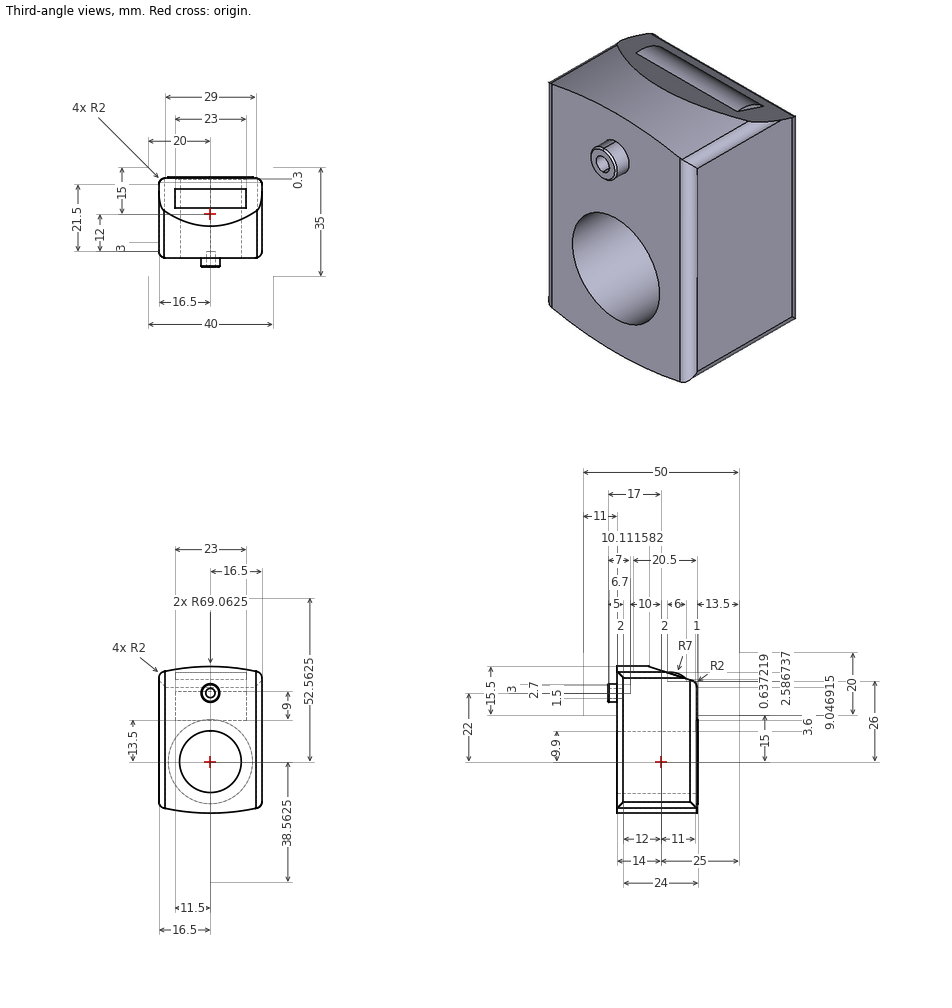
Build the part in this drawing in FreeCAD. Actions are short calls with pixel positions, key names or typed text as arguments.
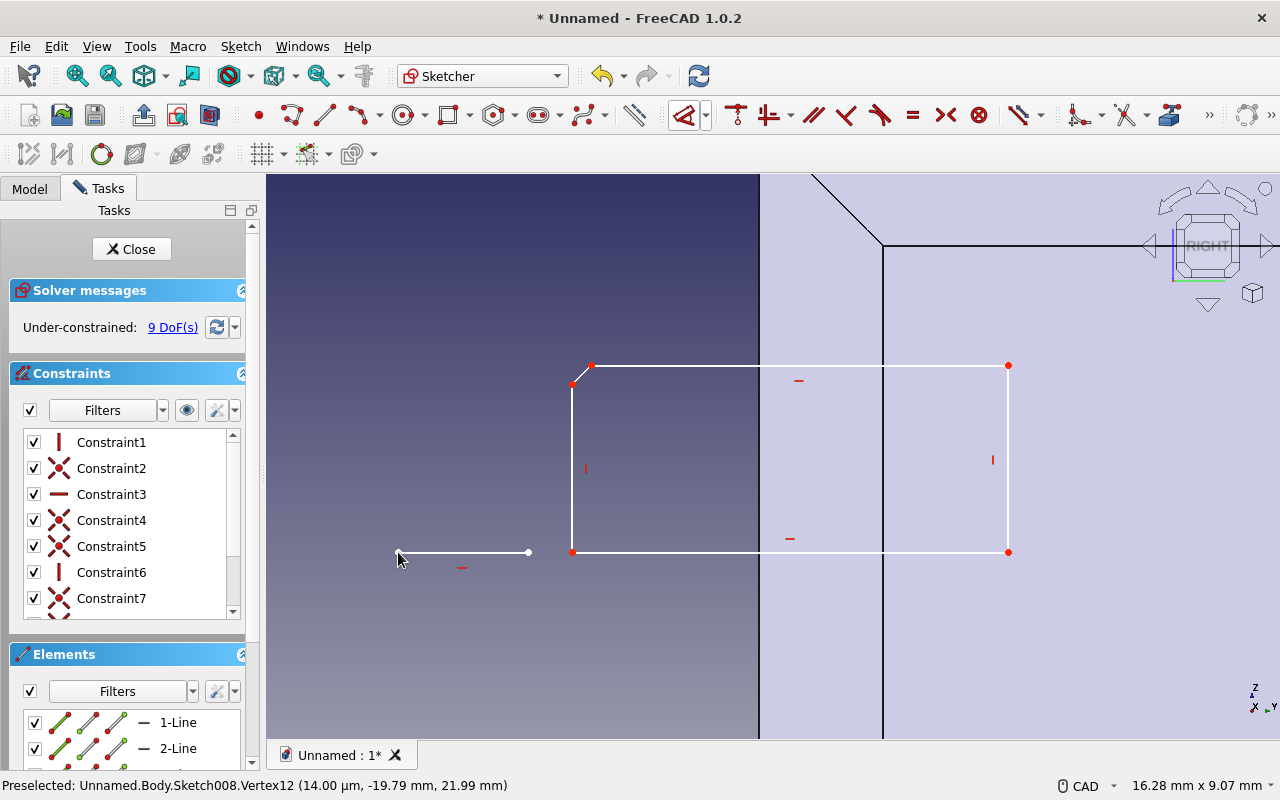
click(489, 553)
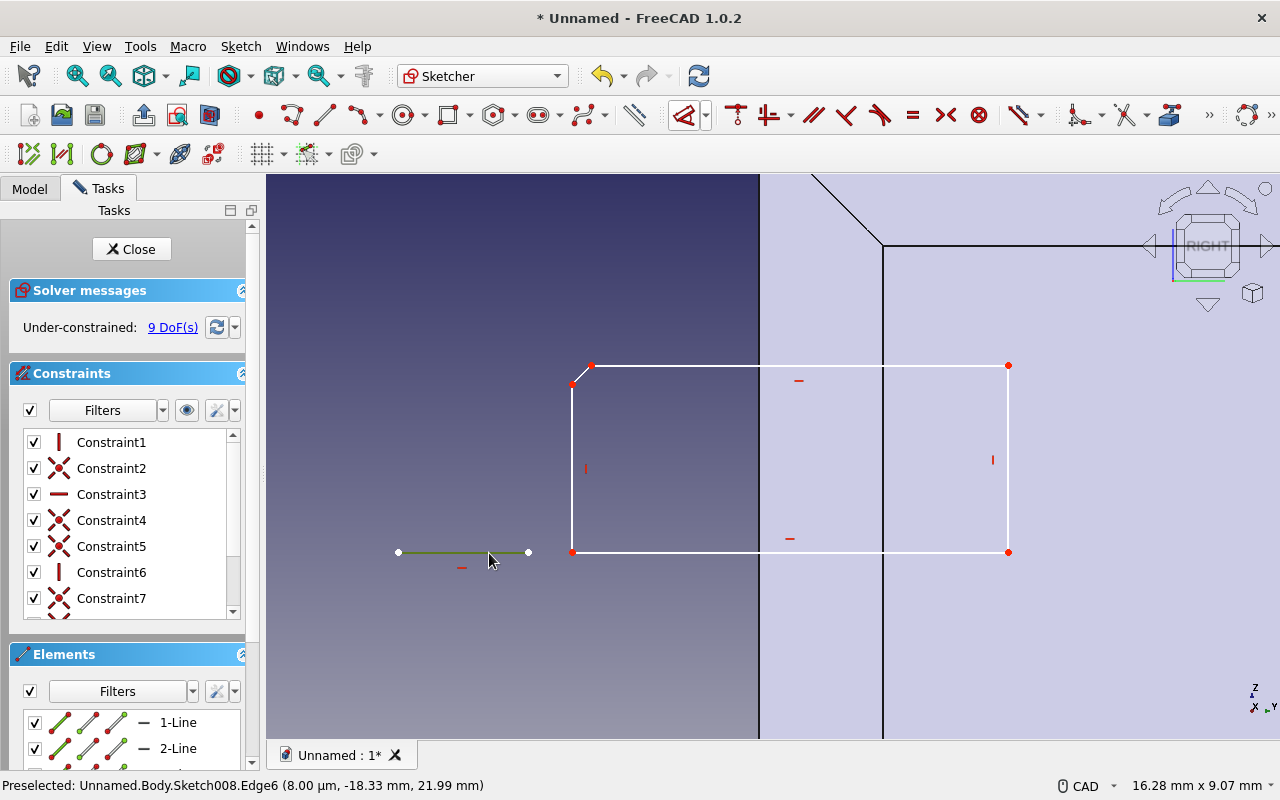
click(635, 116)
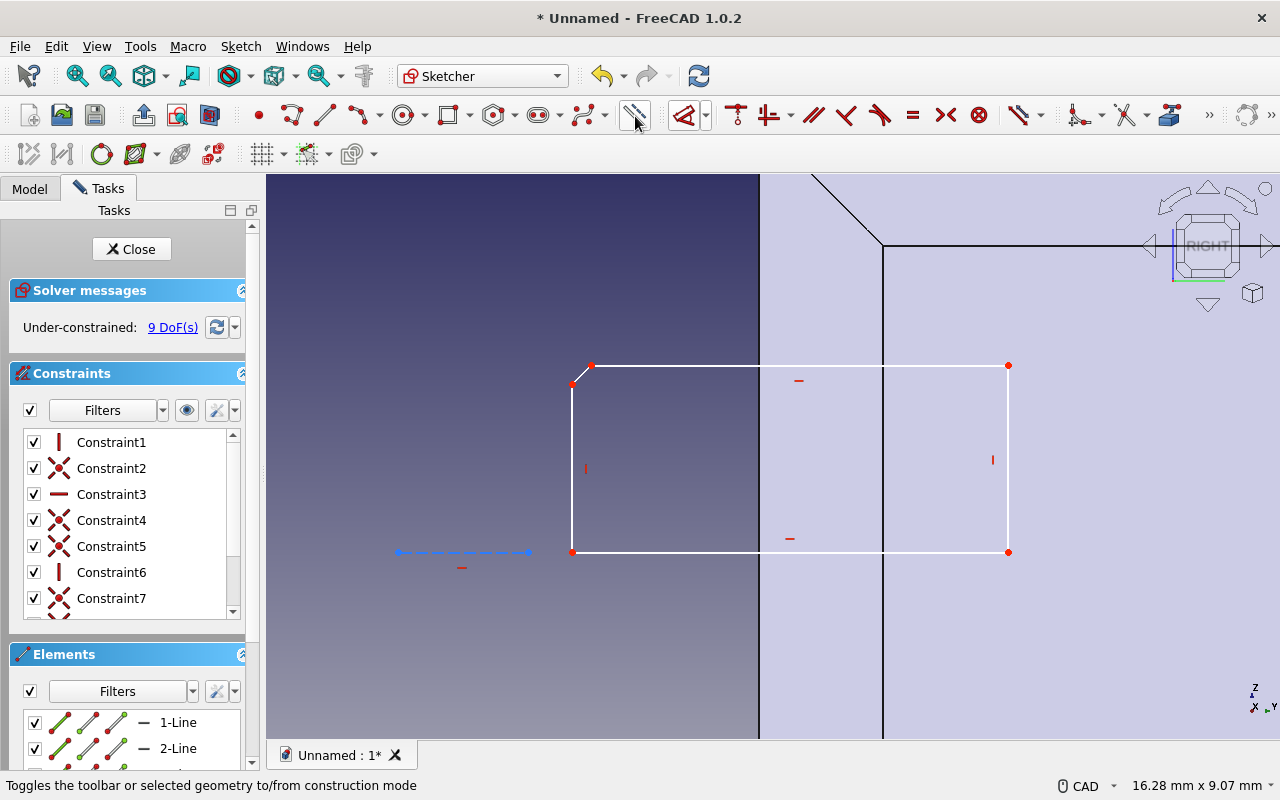
click(1008, 497)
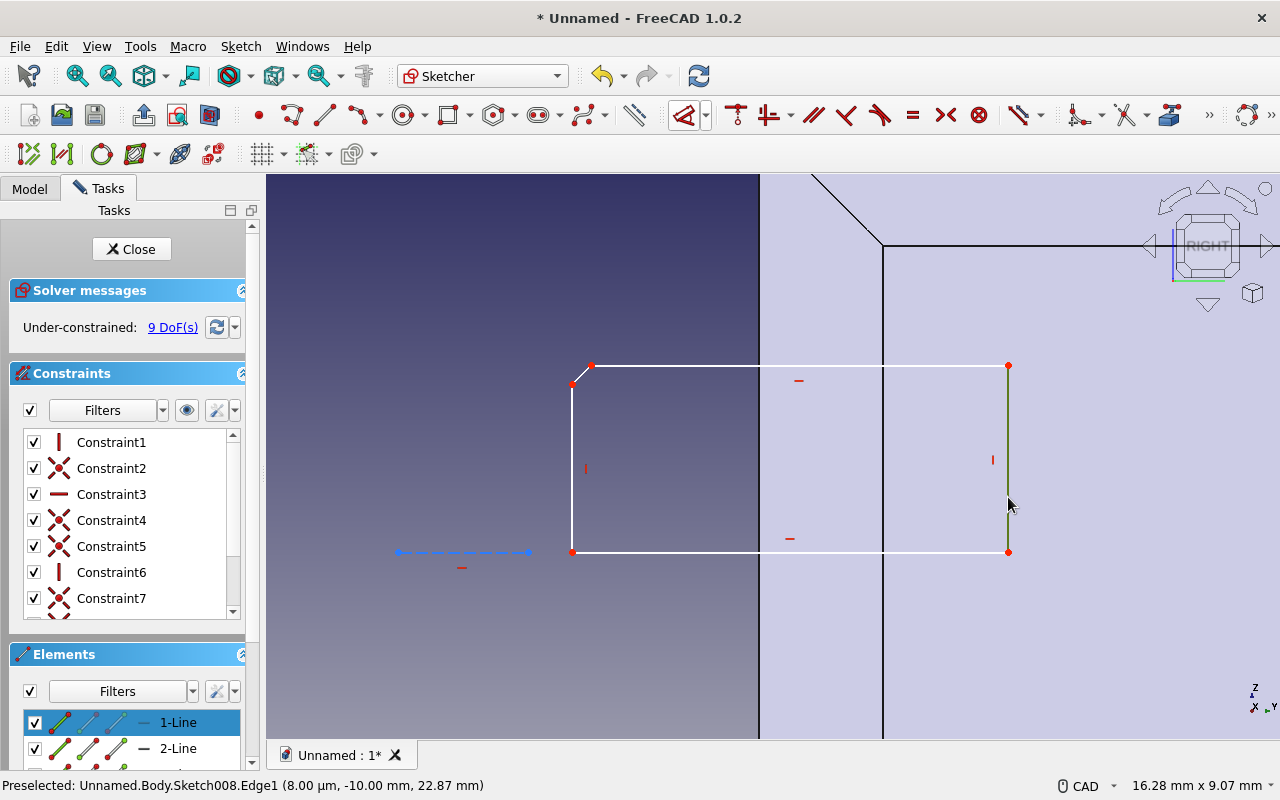
click(706, 116)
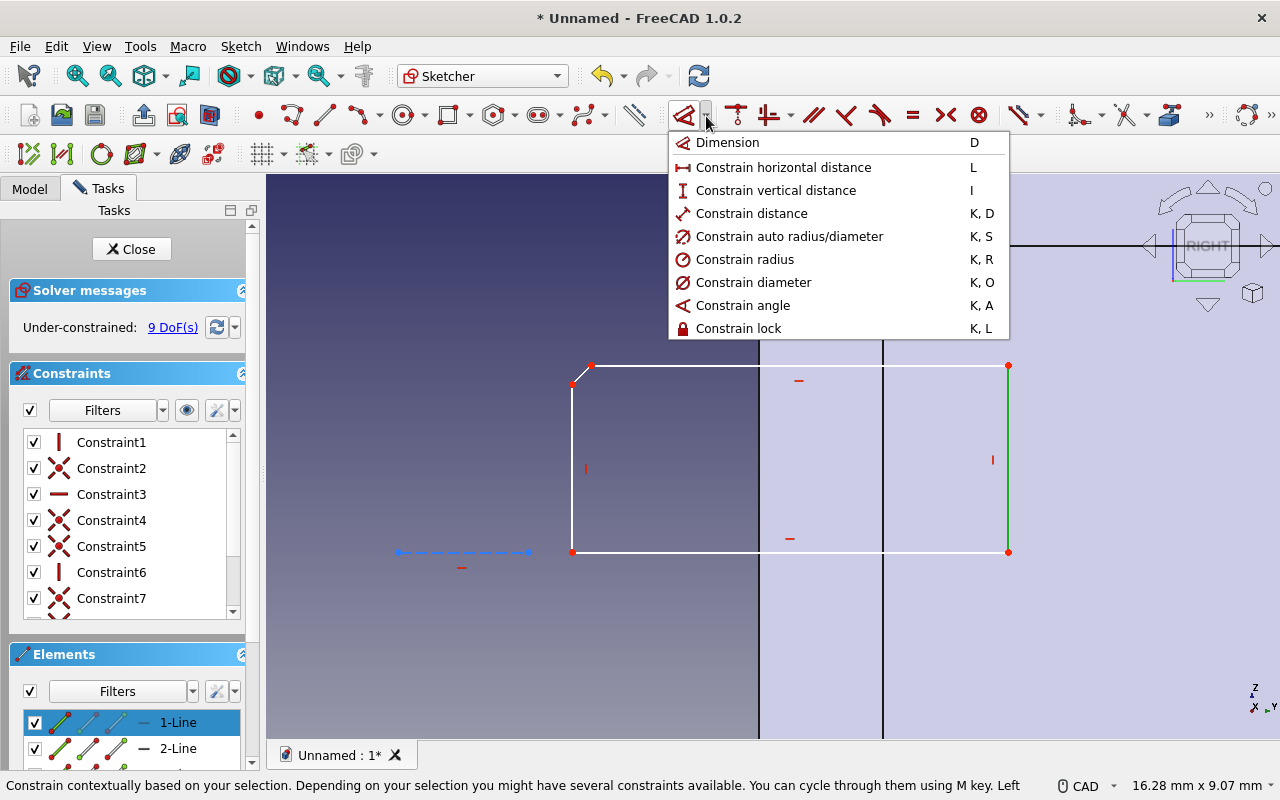
click(839, 190)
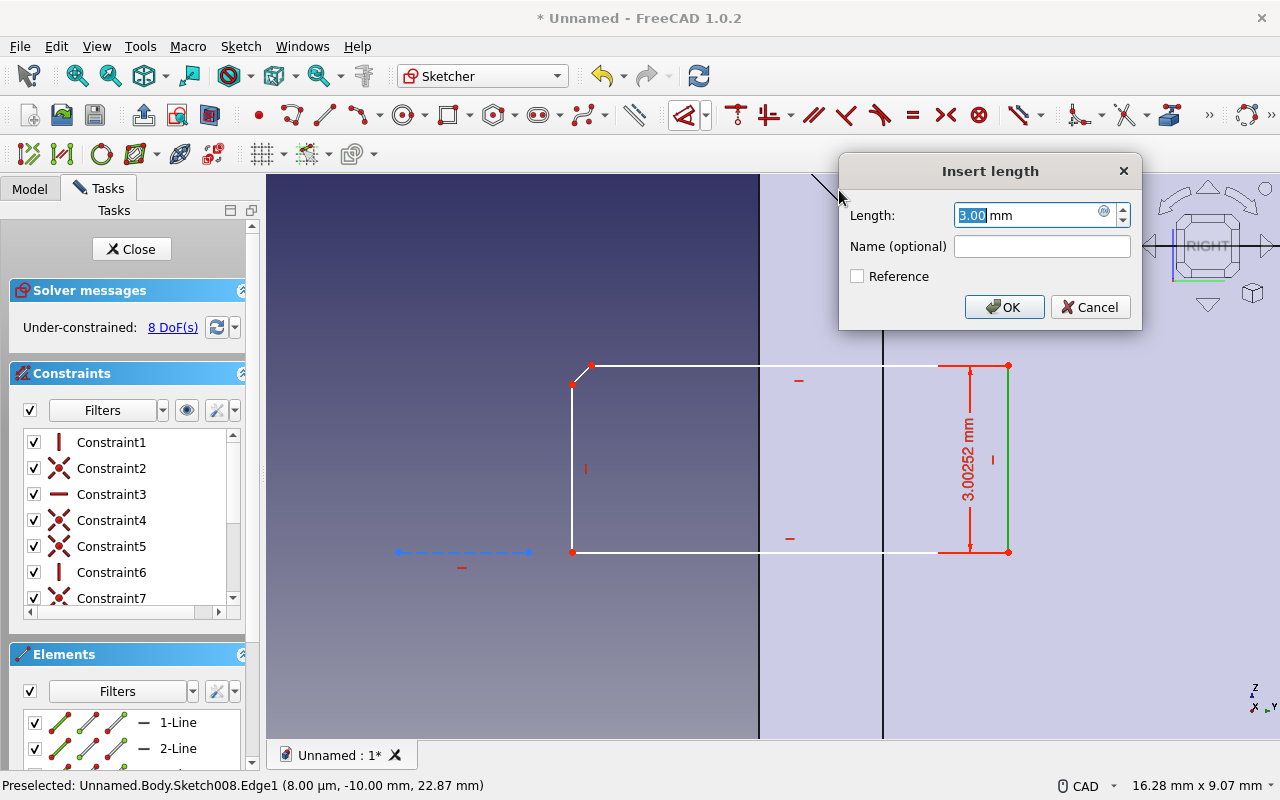
text(3)
key(Return)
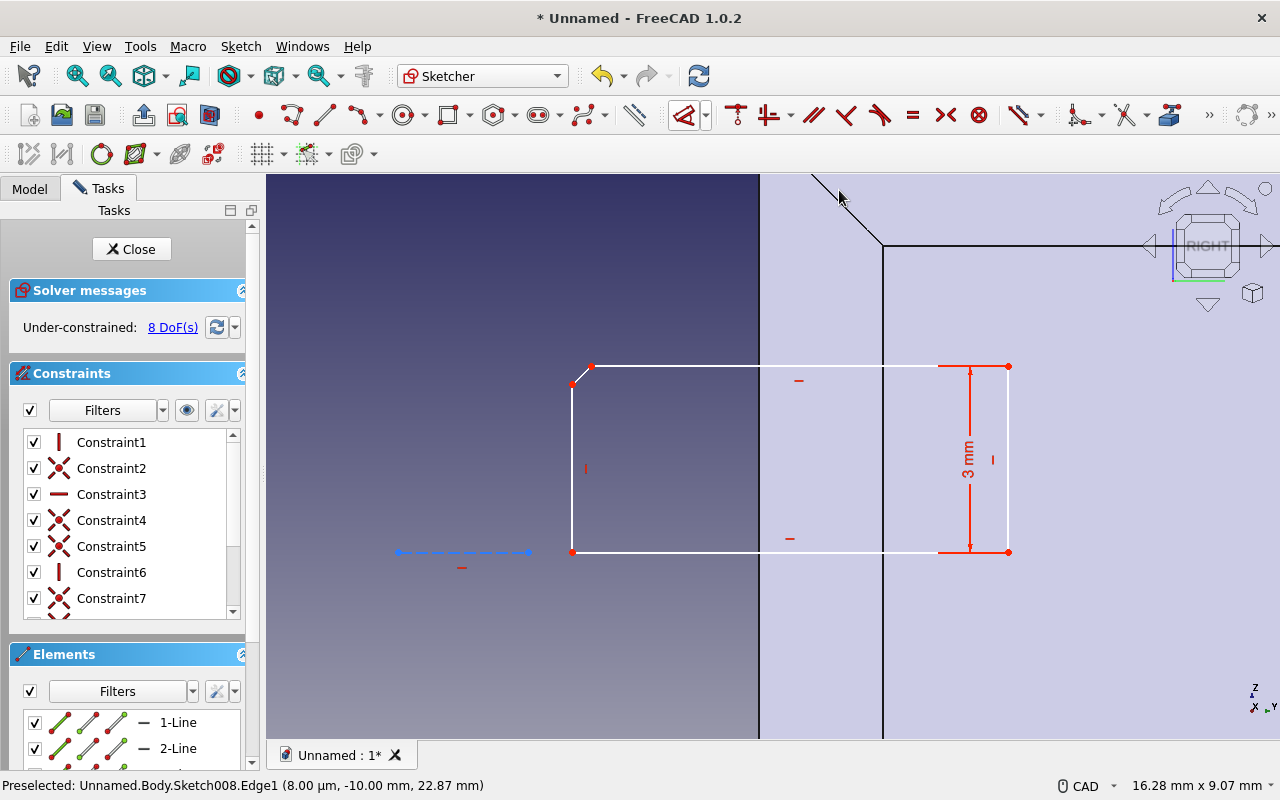
click(703, 553)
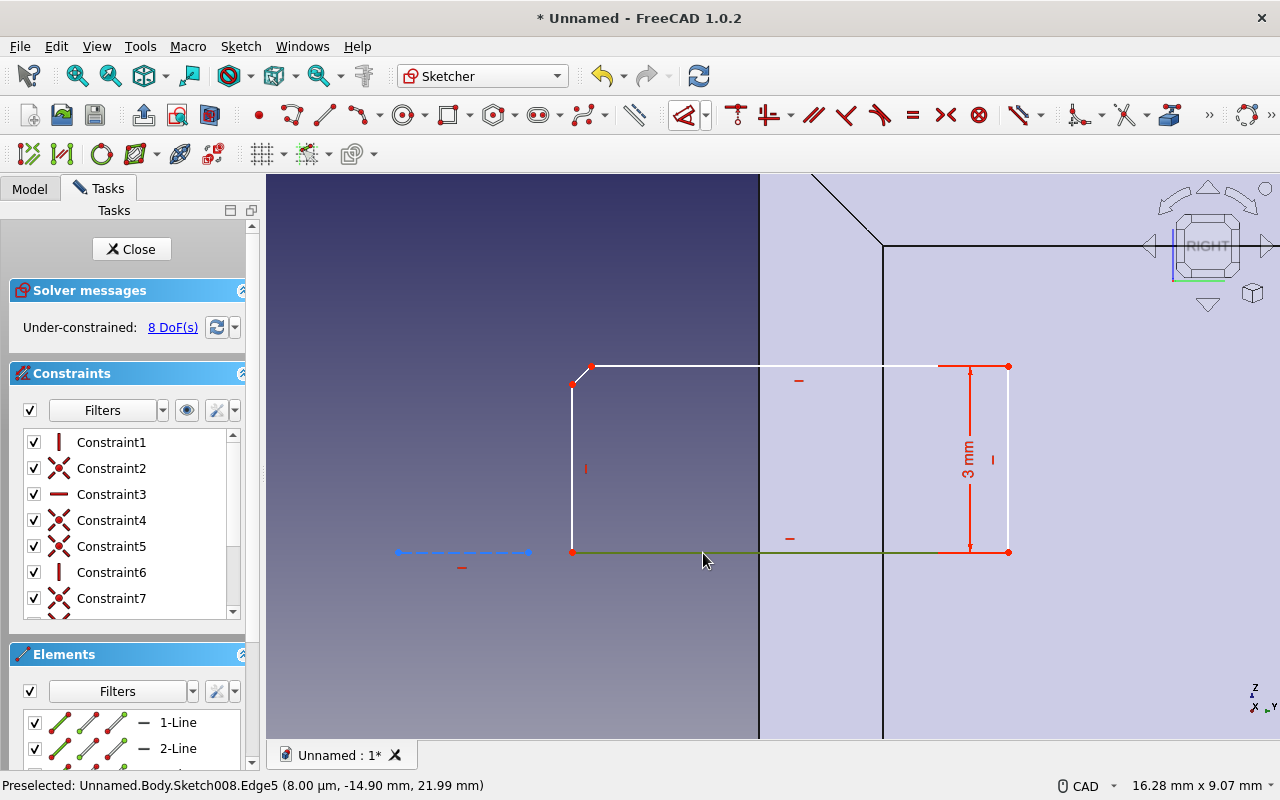
click(706, 116)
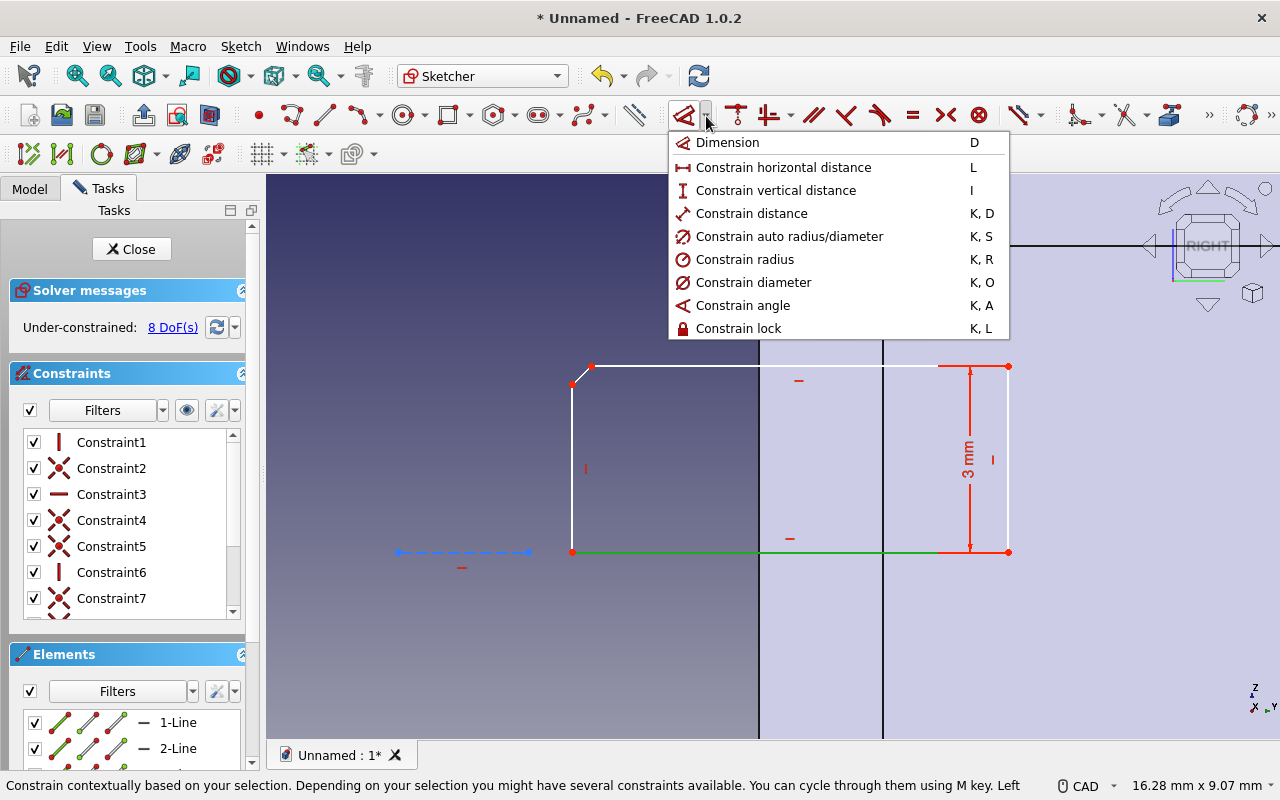
click(839, 168)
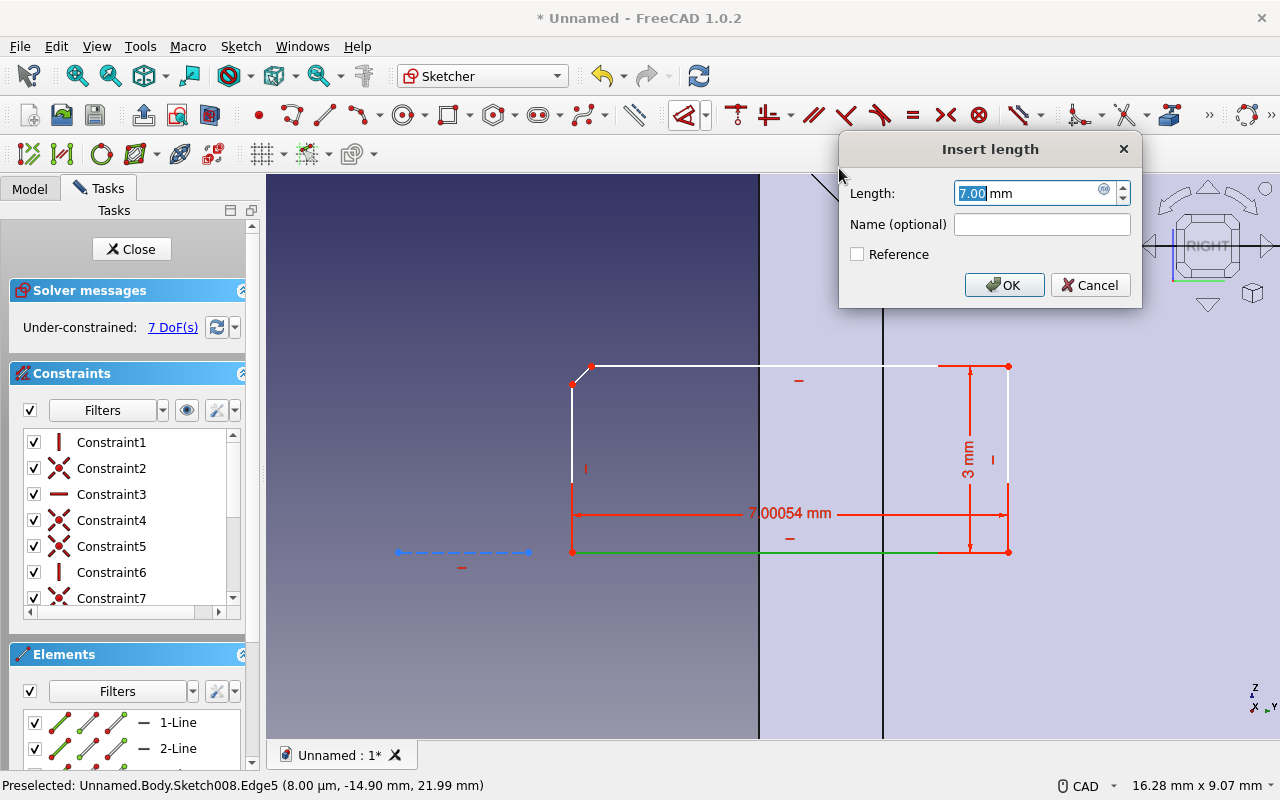
text(7)
key(Return)